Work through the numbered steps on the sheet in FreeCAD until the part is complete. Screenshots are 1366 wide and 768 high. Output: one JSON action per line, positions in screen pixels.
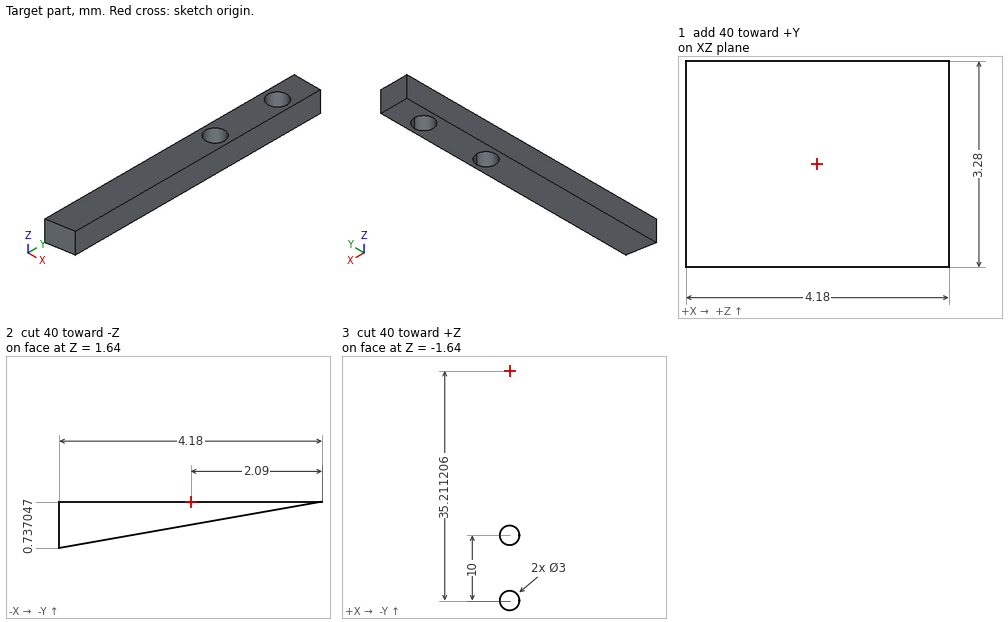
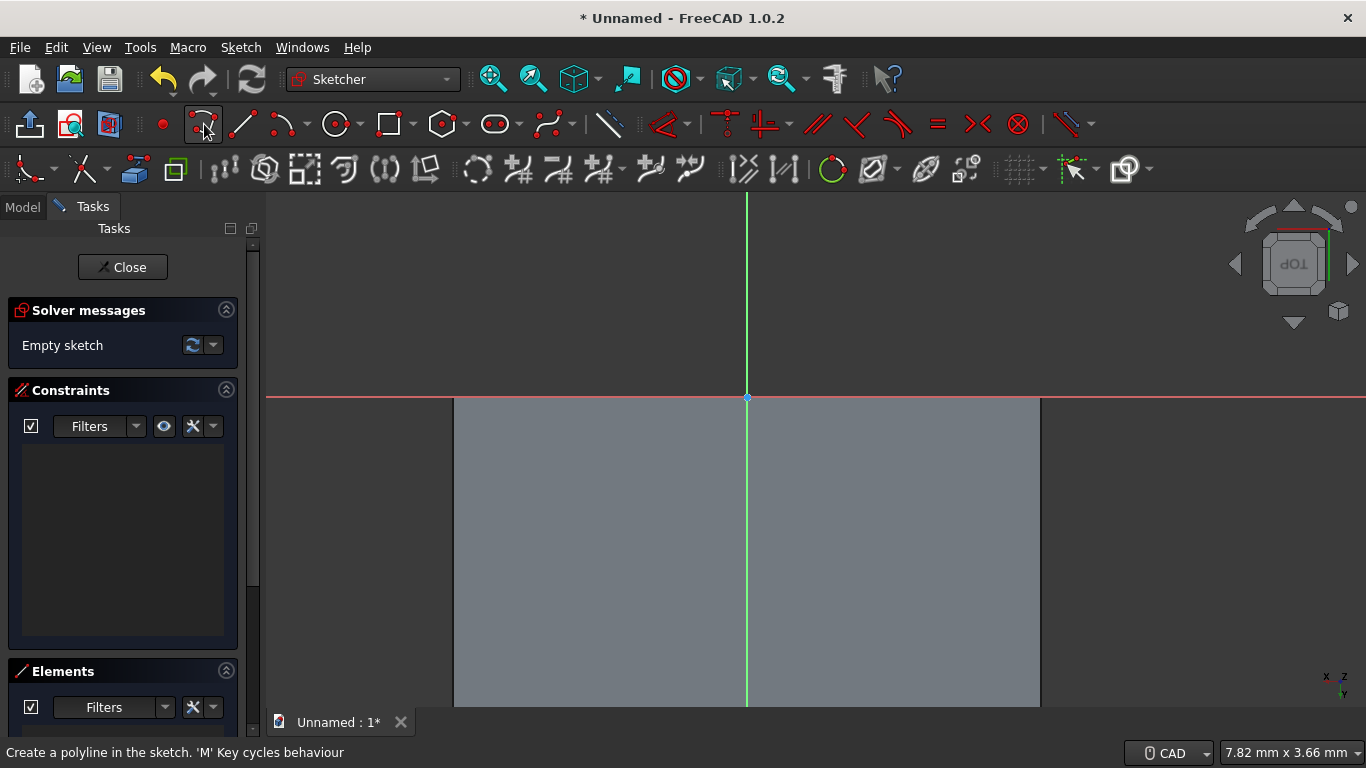
{"action": "left_click", "coordinate": [1041, 397]}
{"action": "left_click", "coordinate": [453, 406]}
{"action": "left_click", "coordinate": [453, 501]}
{"action": "left_click", "coordinate": [1041, 397]}
{"action": "key", "text": "Escape"}
{"action": "key", "text": "Escape"}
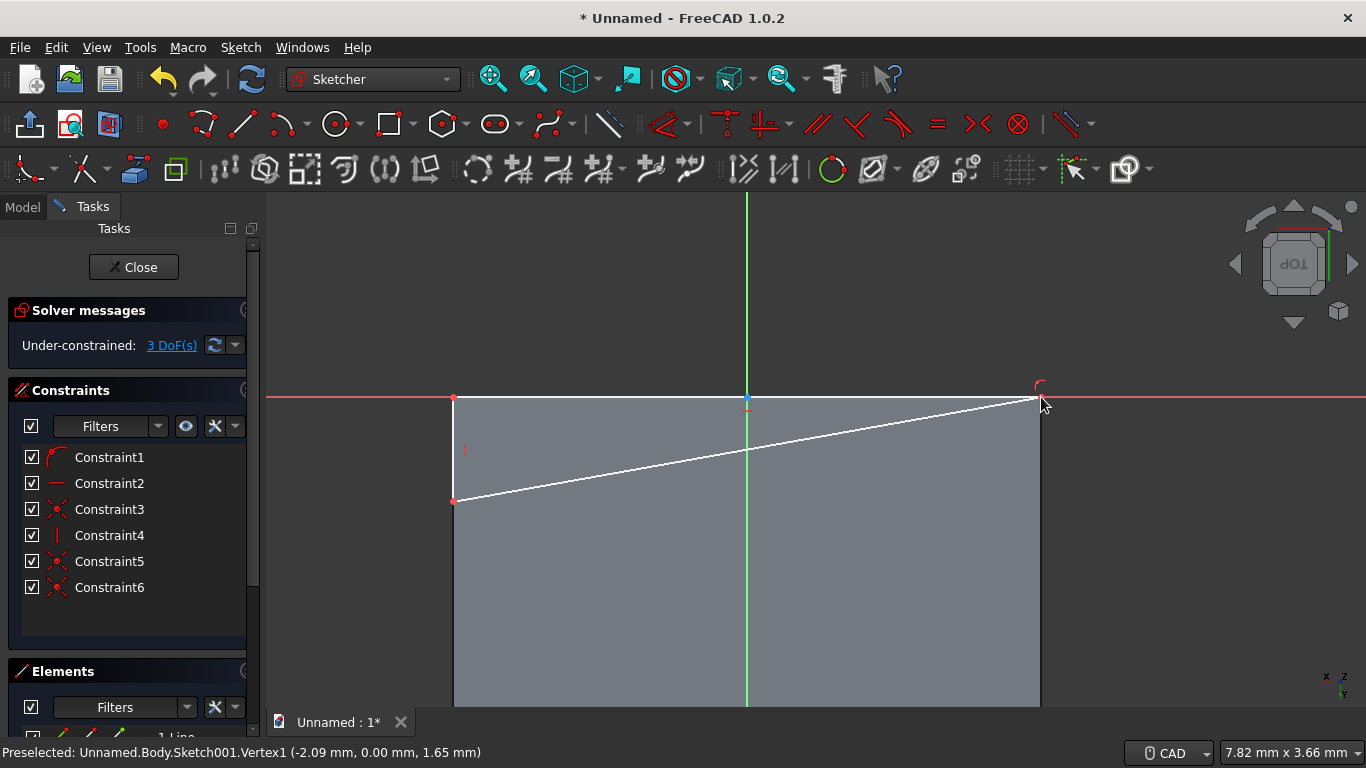
{"action": "left_click", "coordinate": [664, 124]}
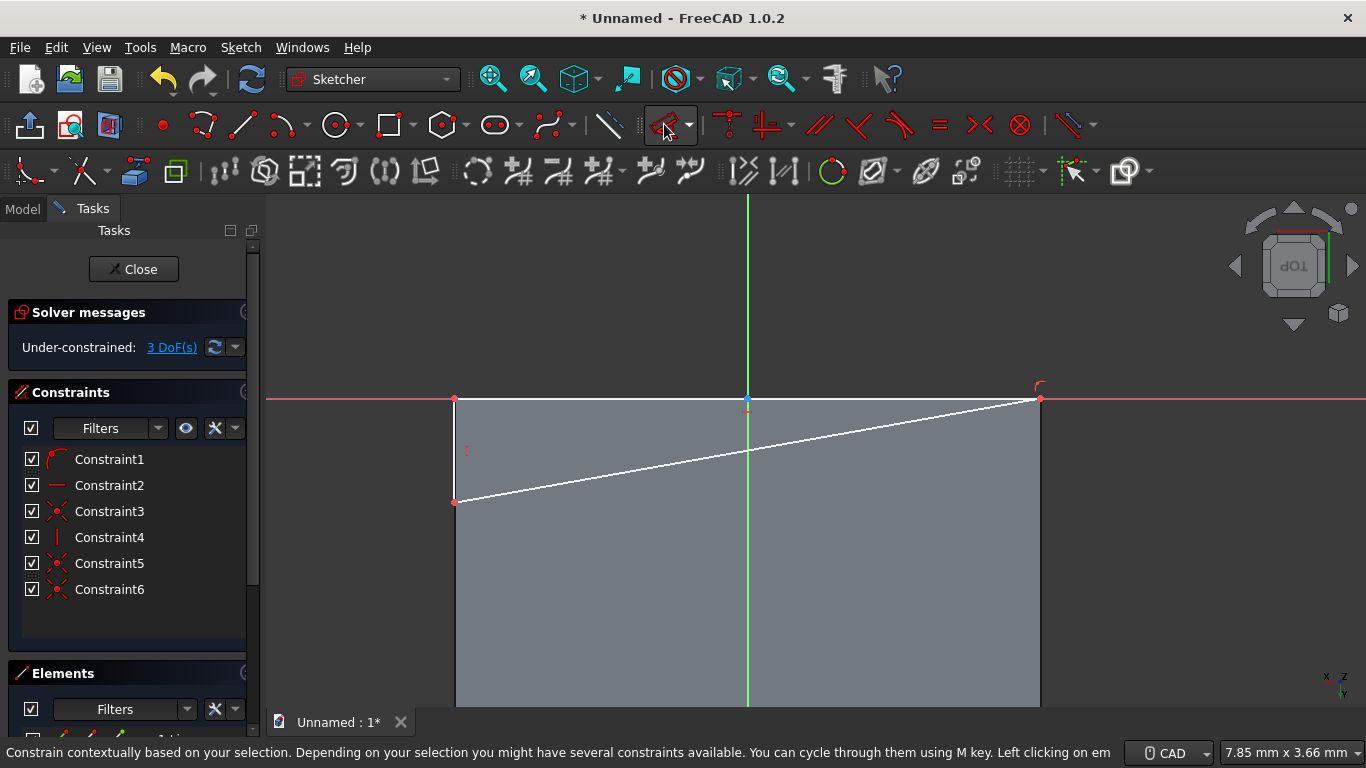
{"action": "left_click", "coordinate": [864, 399]}
{"action": "left_click", "coordinate": [613, 365]}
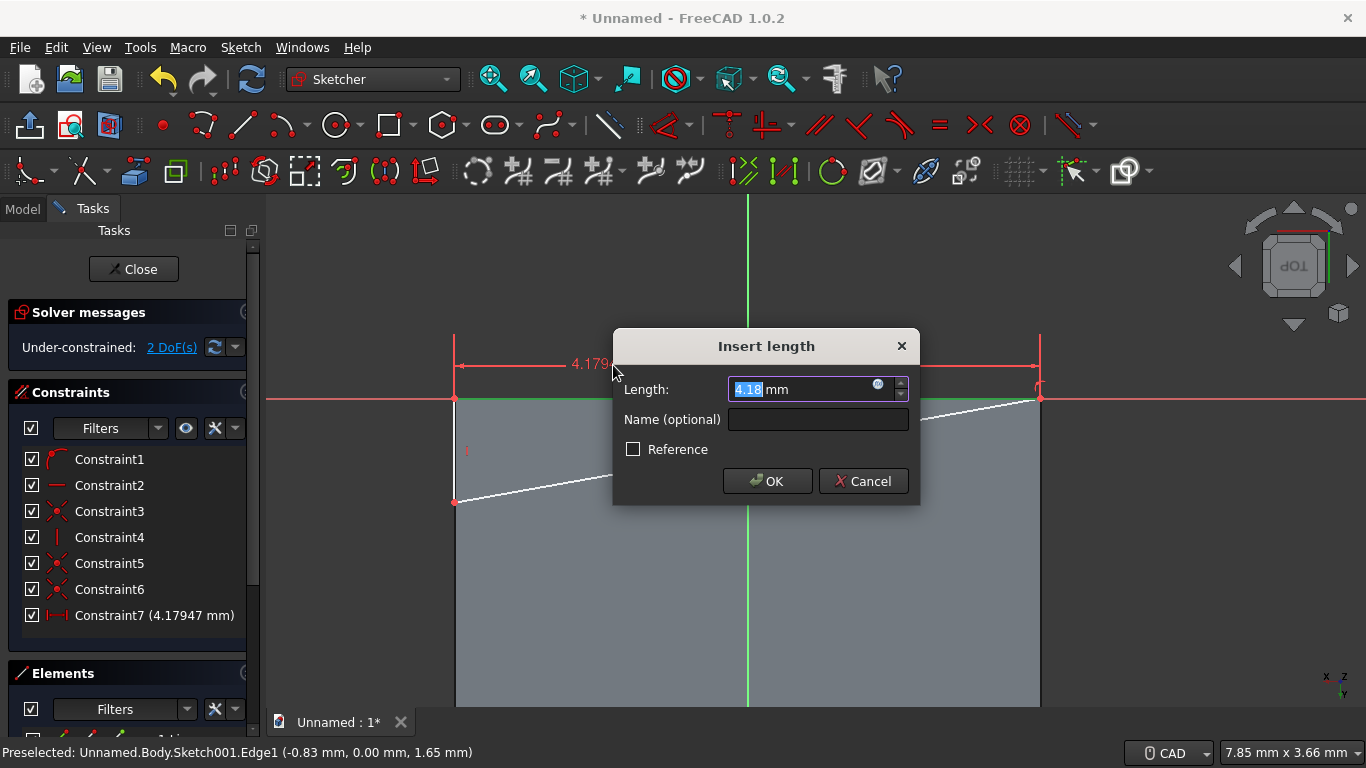
{"action": "type", "text": "4.18"}
{"action": "key", "text": "Return"}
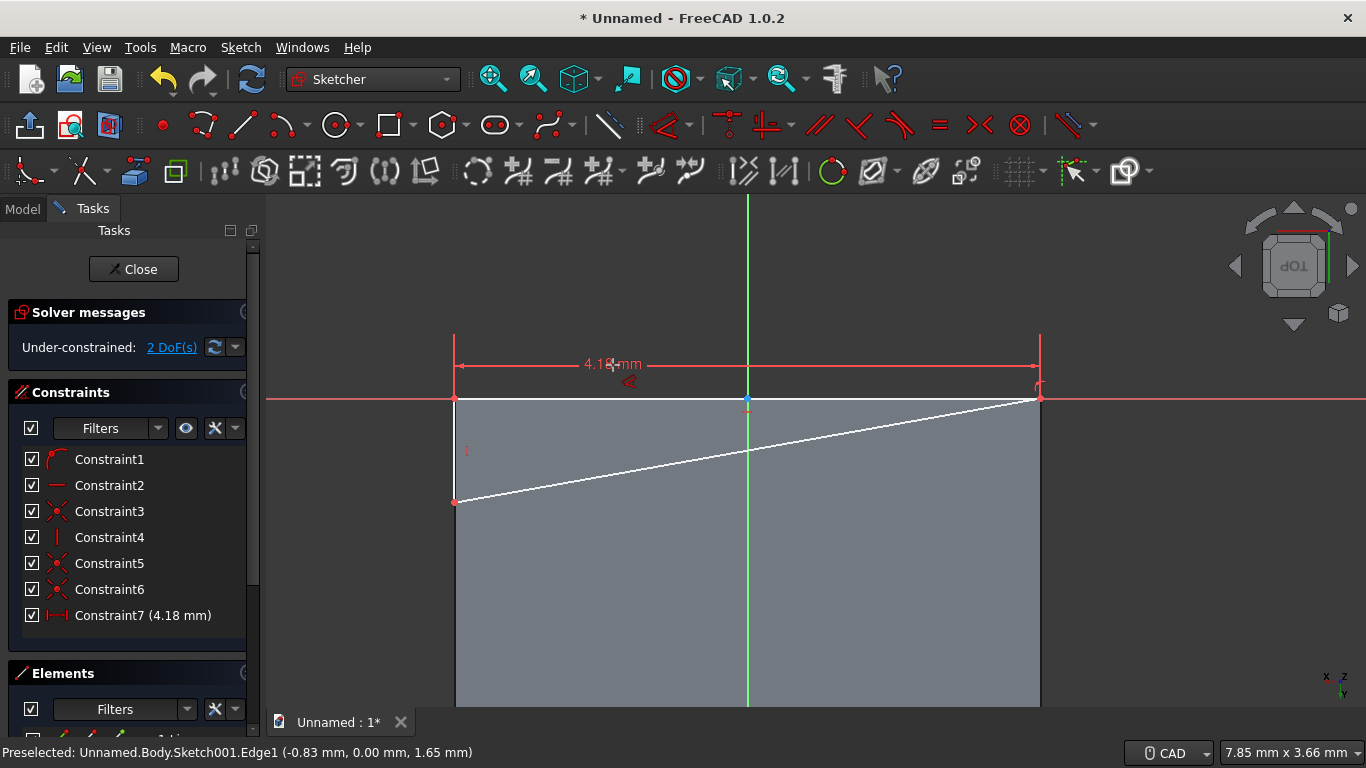
{"action": "left_click", "coordinate": [1040, 399]}
{"action": "left_click", "coordinate": [894, 365]}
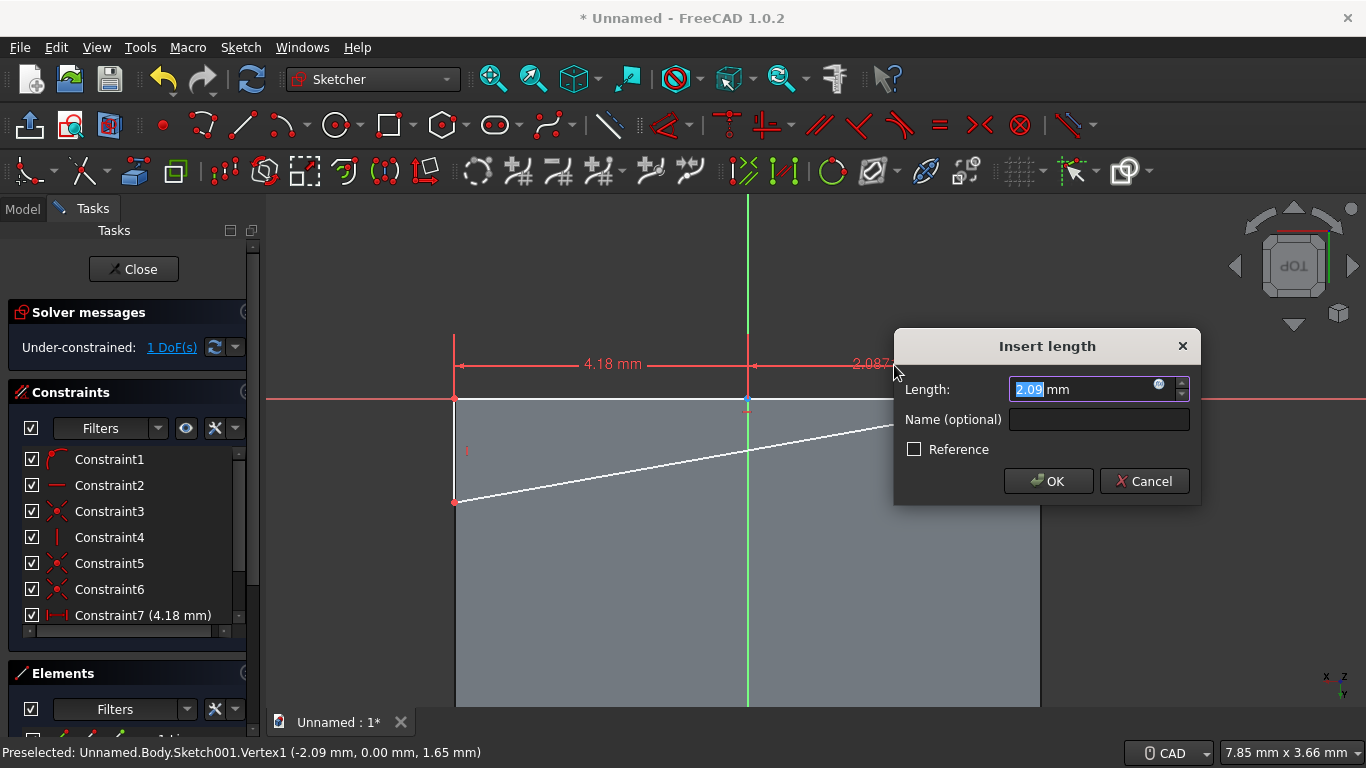
{"action": "type", "text": "2.09"}
{"action": "key", "text": "Return"}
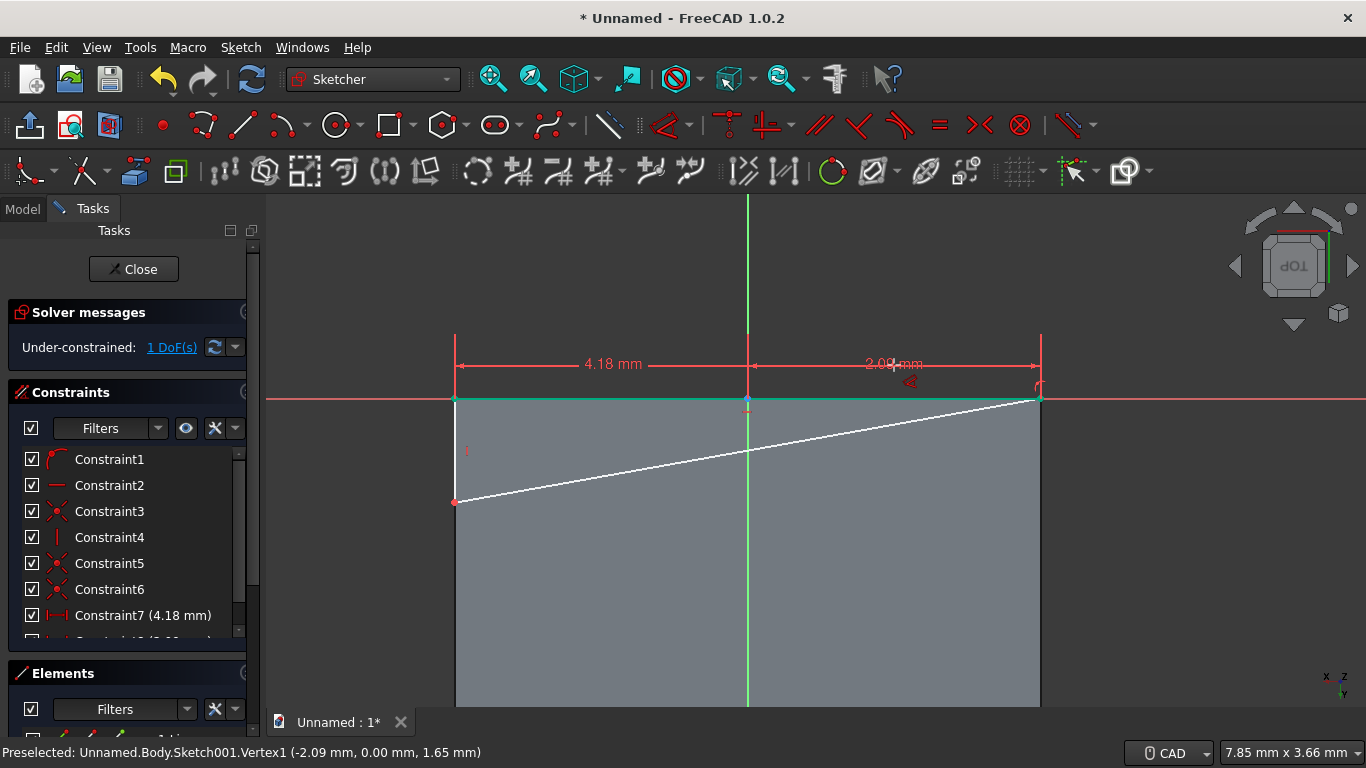
{"action": "left_click", "coordinate": [455, 430]}
{"action": "left_click", "coordinate": [421, 451]}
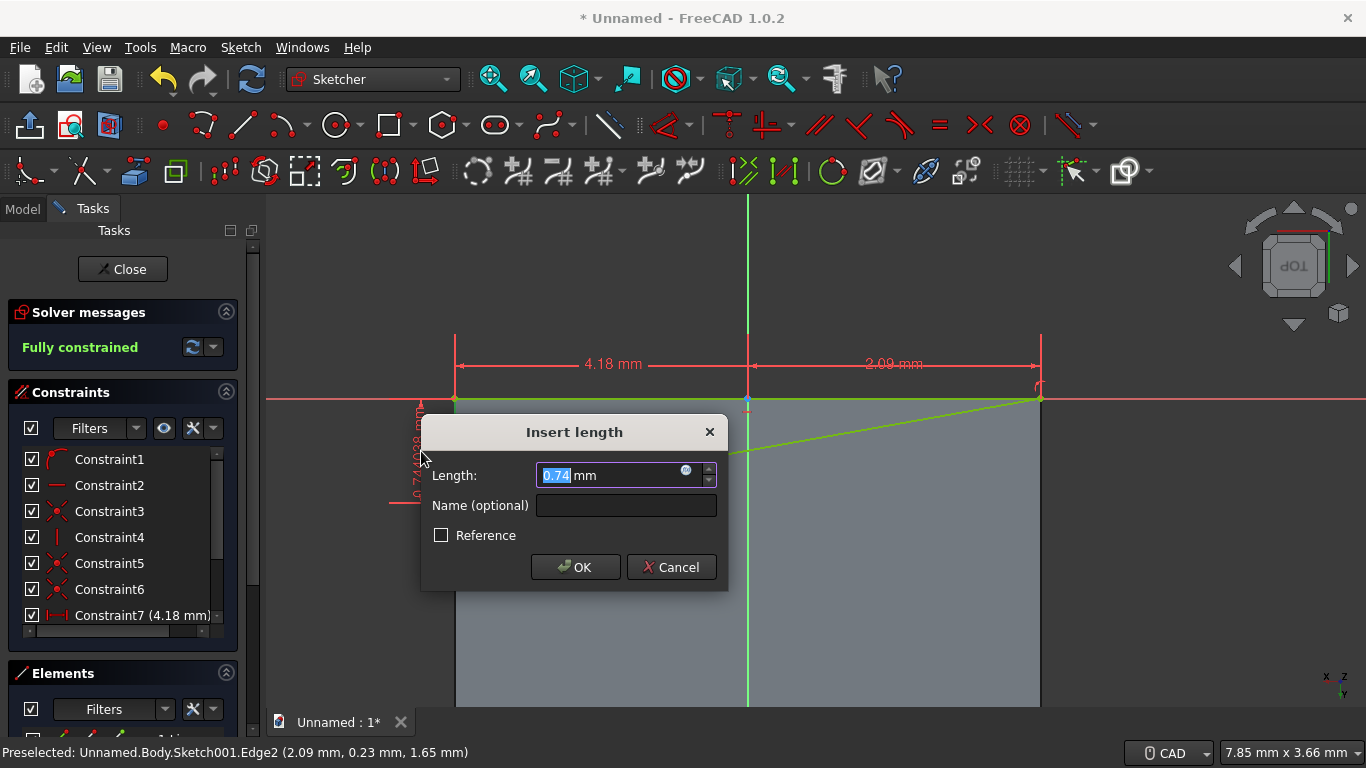
{"action": "type", "text": "0.737047"}
{"action": "key", "text": "Return"}
{"action": "key", "text": "Escape"}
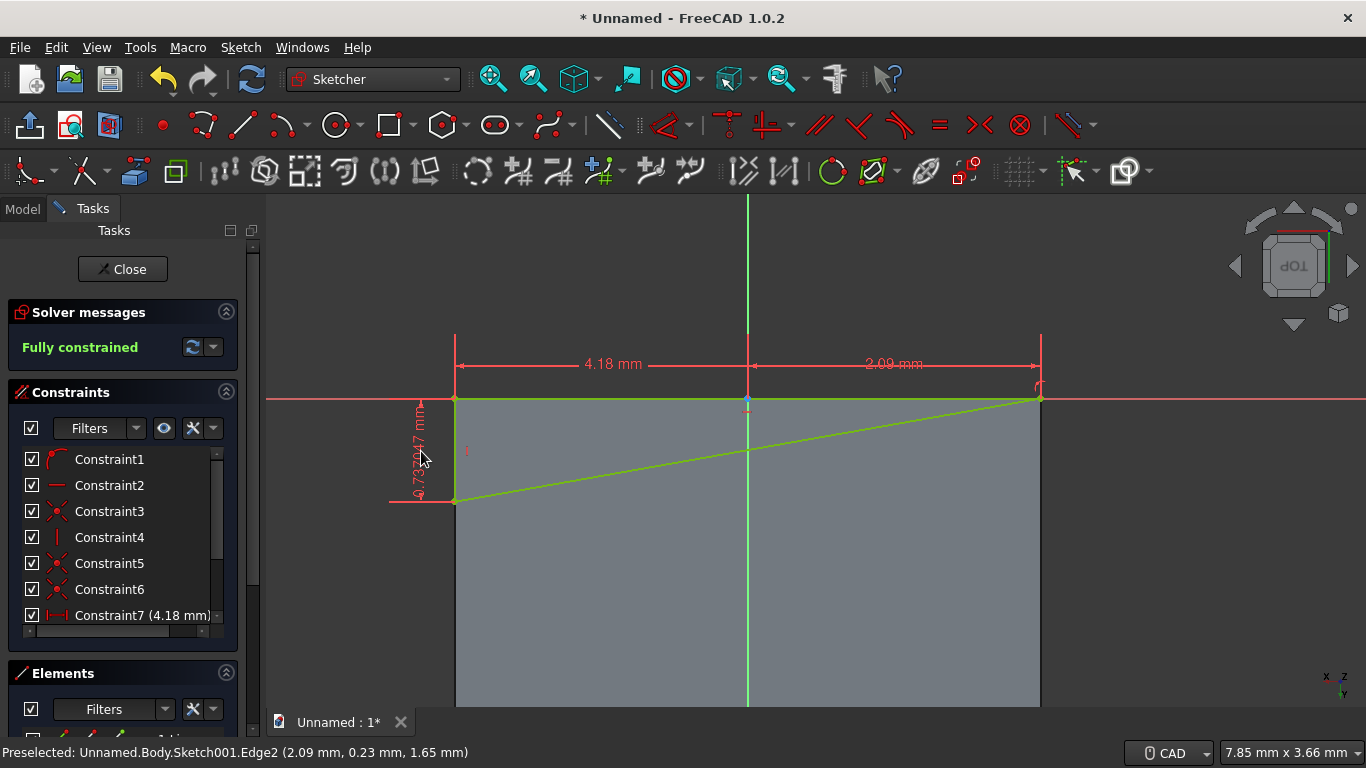
{"action": "left_click", "coordinate": [123, 269]}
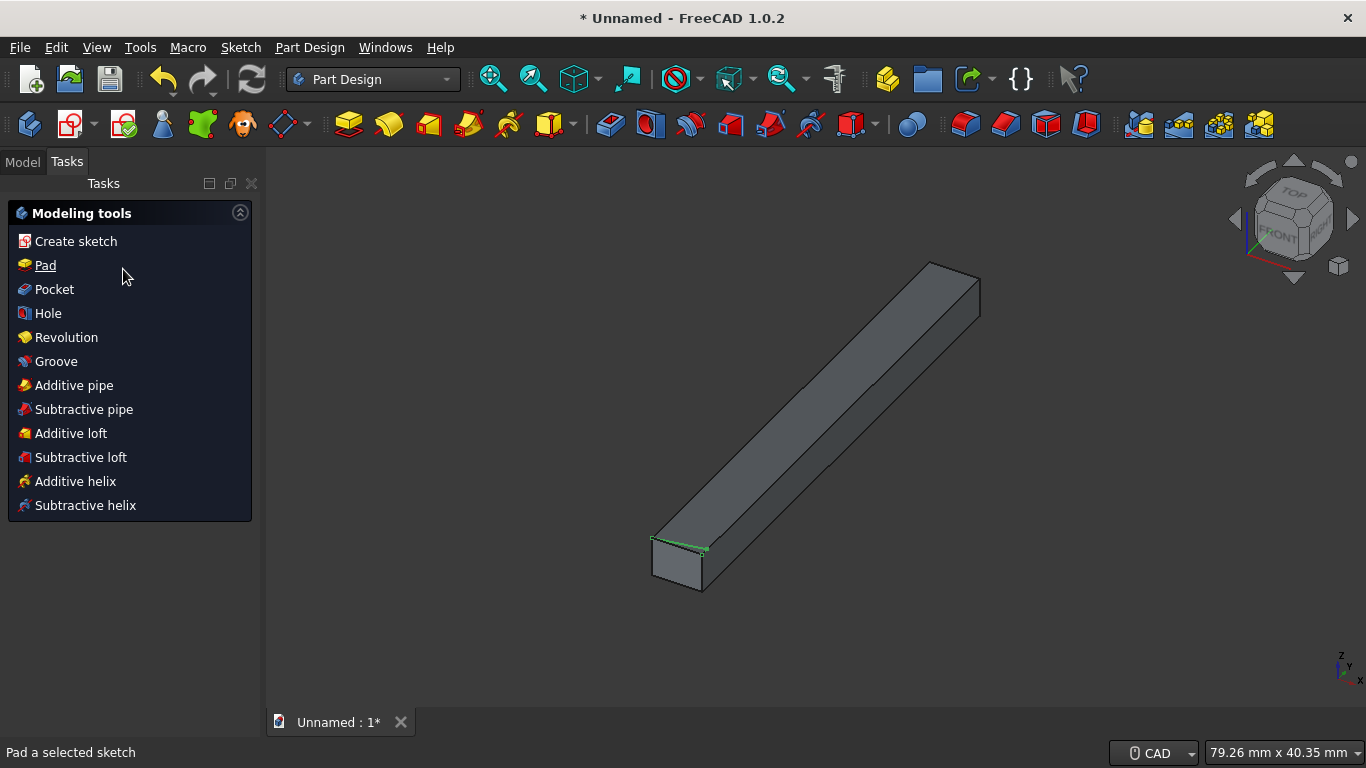
{"action": "left_click", "coordinate": [612, 124]}